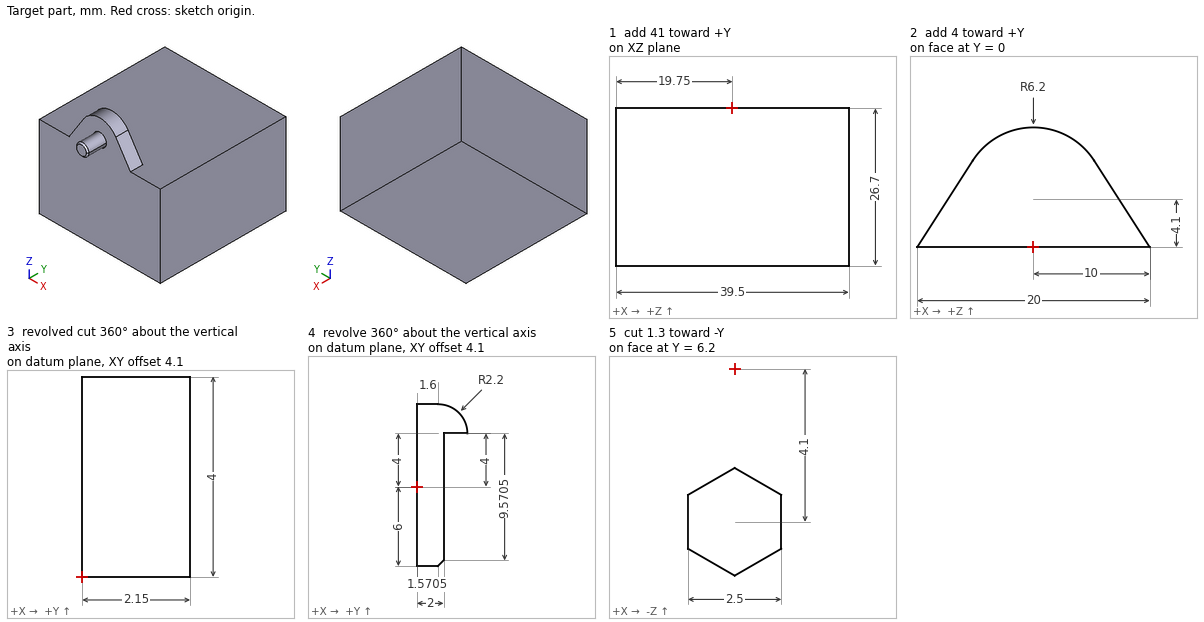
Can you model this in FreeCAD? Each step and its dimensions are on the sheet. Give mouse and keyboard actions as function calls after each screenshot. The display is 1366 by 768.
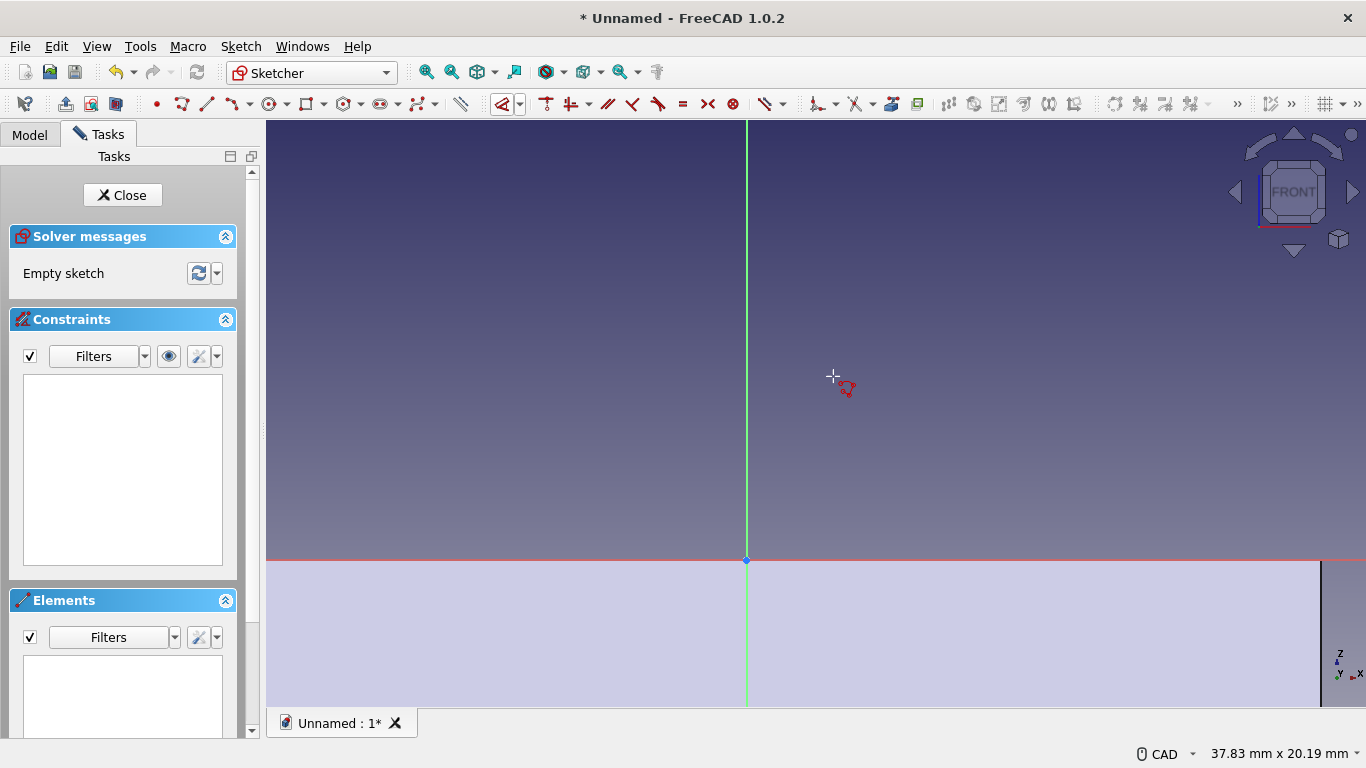
click(898, 343)
click(1038, 560)
click(456, 551)
click(595, 343)
right_click(595, 343)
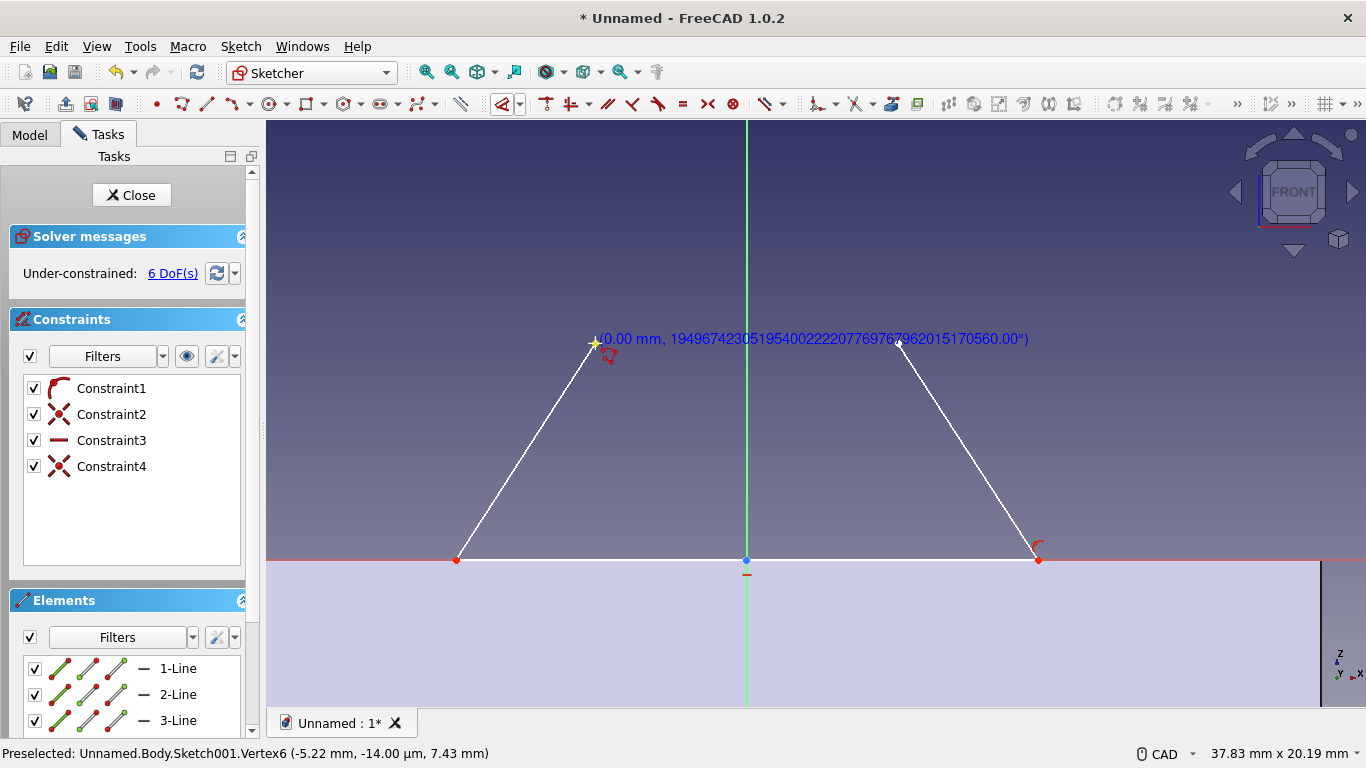
click(232, 104)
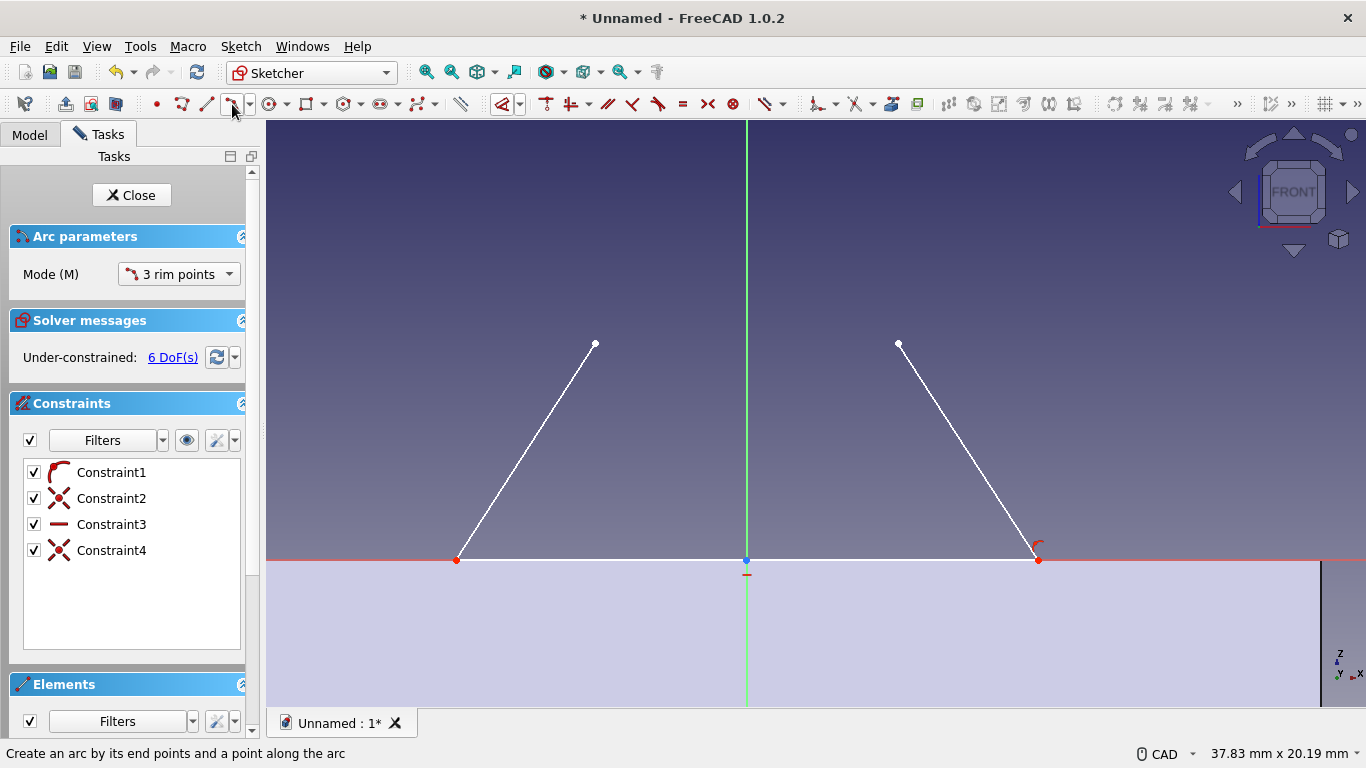
click(595, 344)
click(898, 344)
click(783, 264)
key(Escape)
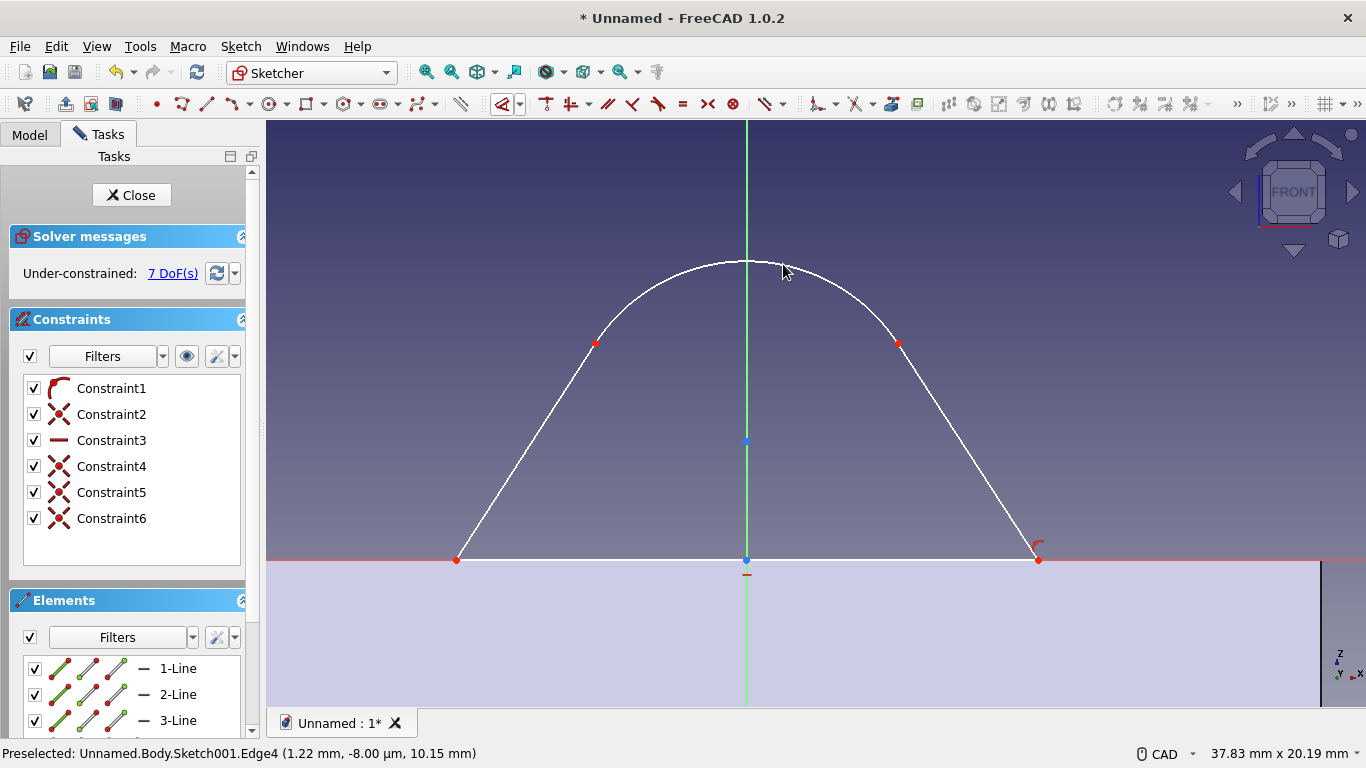
click(940, 409)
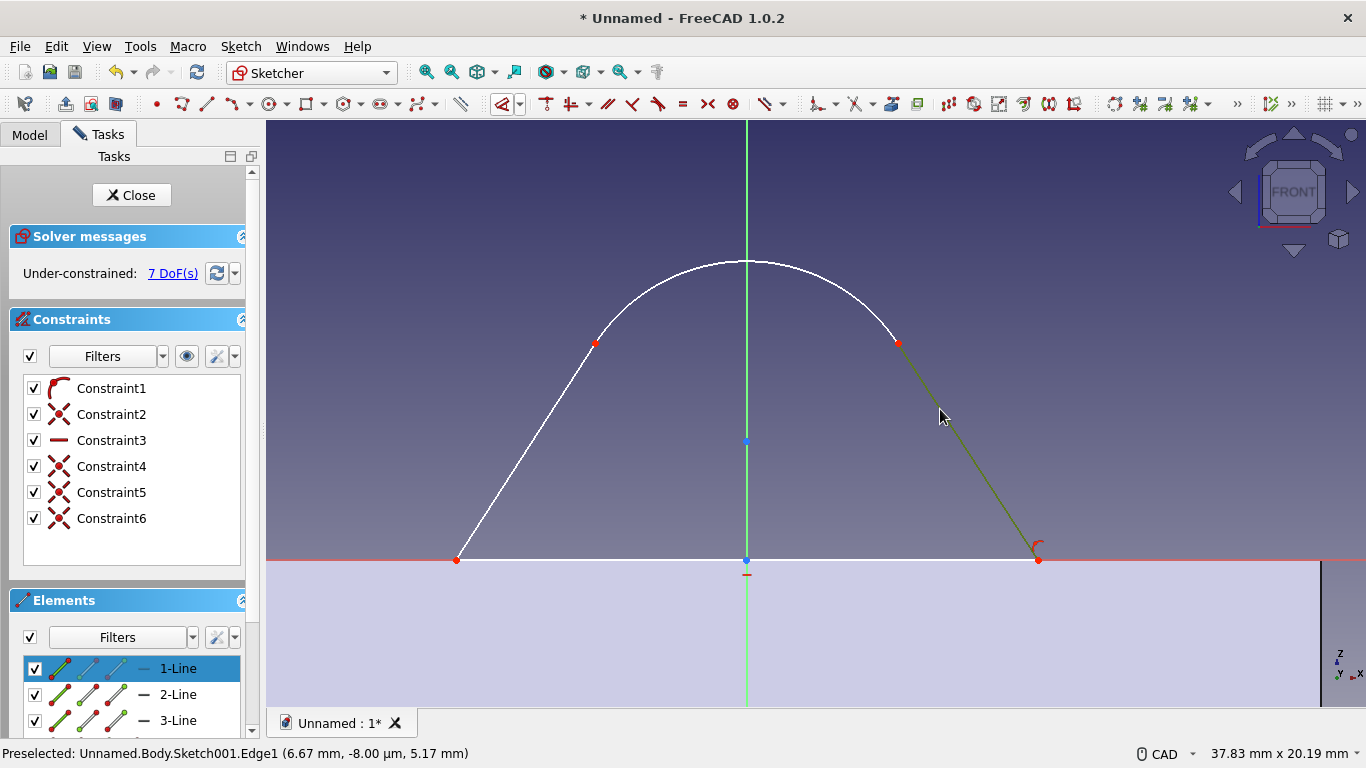
click(817, 275)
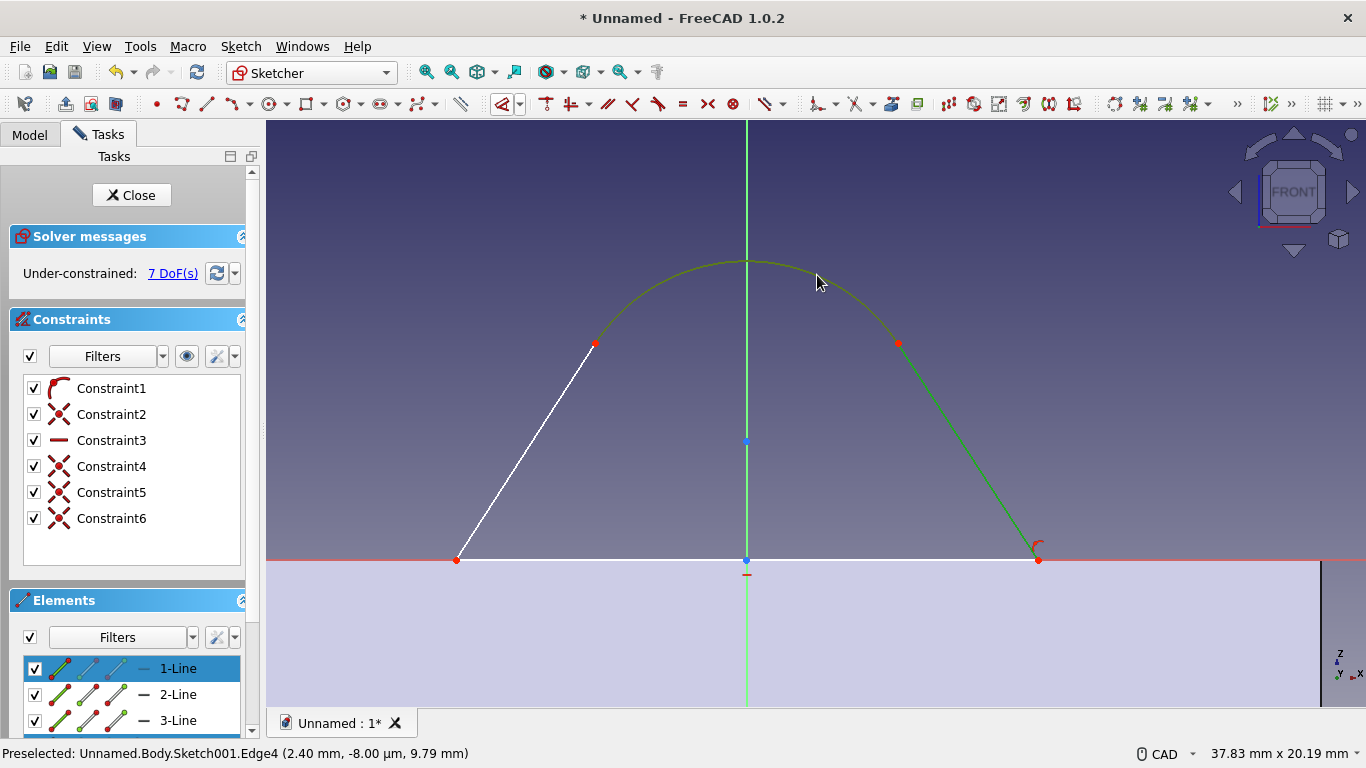
key(t)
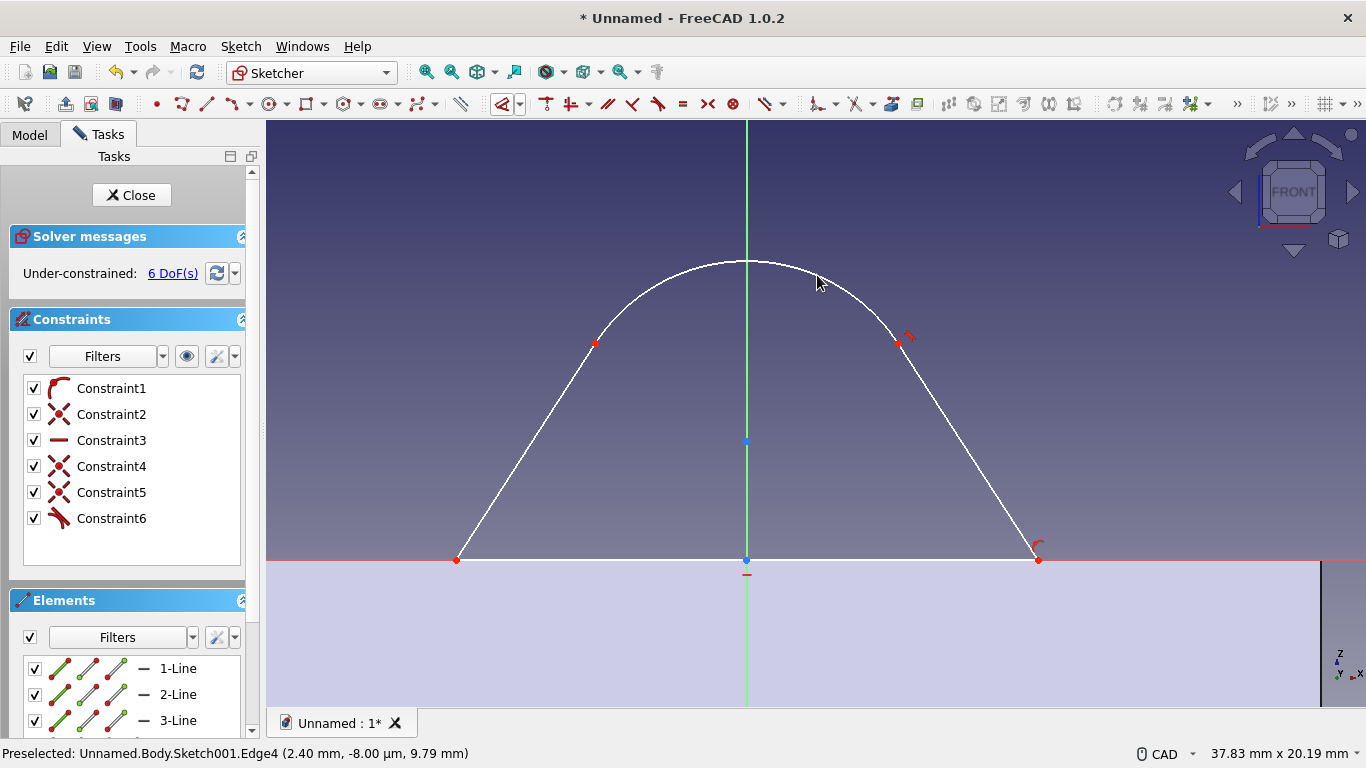
click(498, 495)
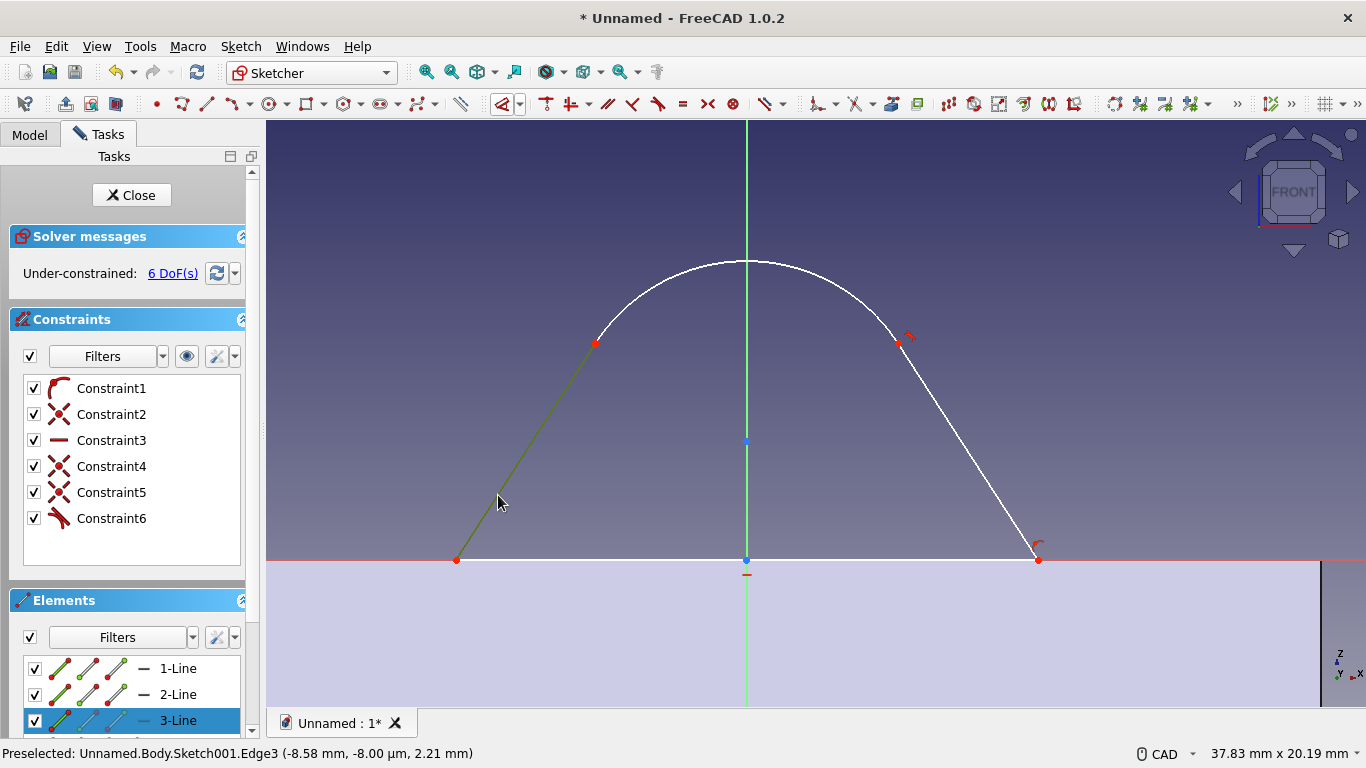
click(816, 275)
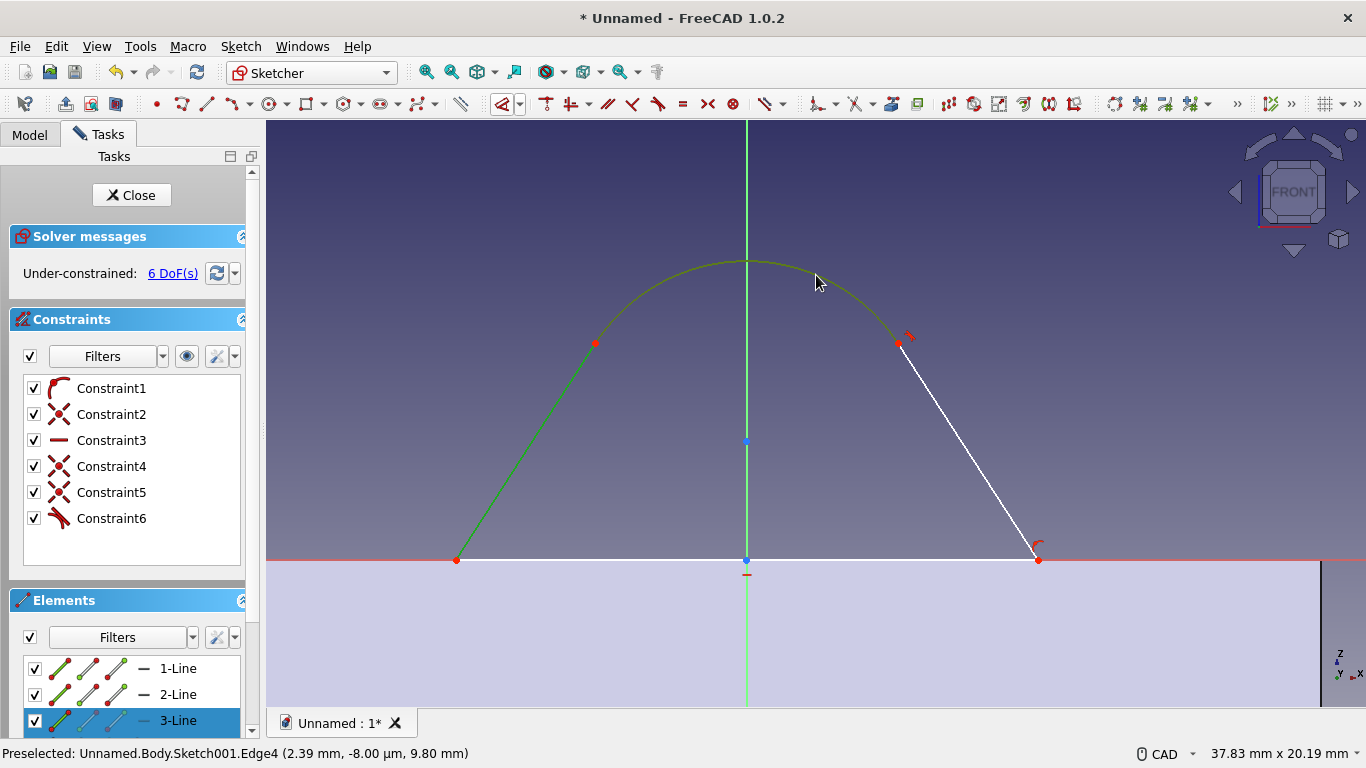
click(658, 104)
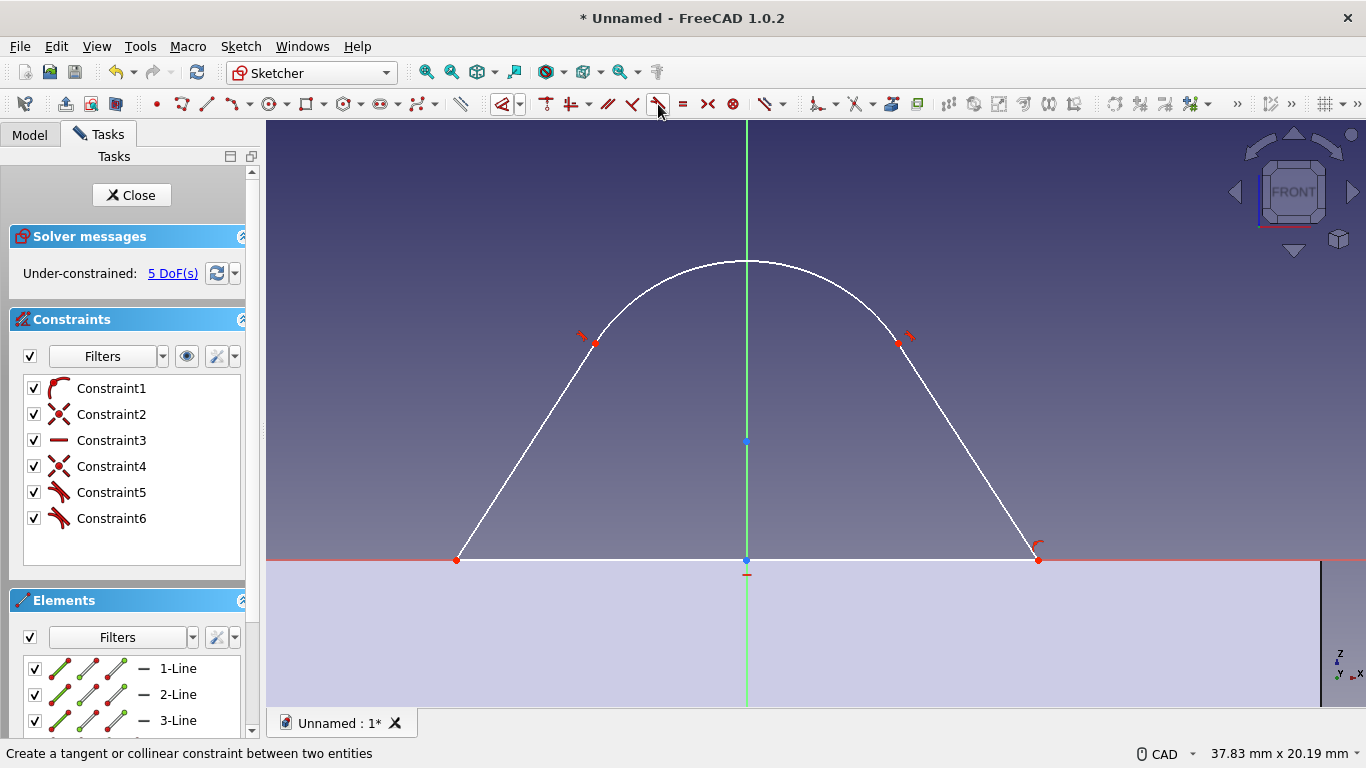
click(747, 441)